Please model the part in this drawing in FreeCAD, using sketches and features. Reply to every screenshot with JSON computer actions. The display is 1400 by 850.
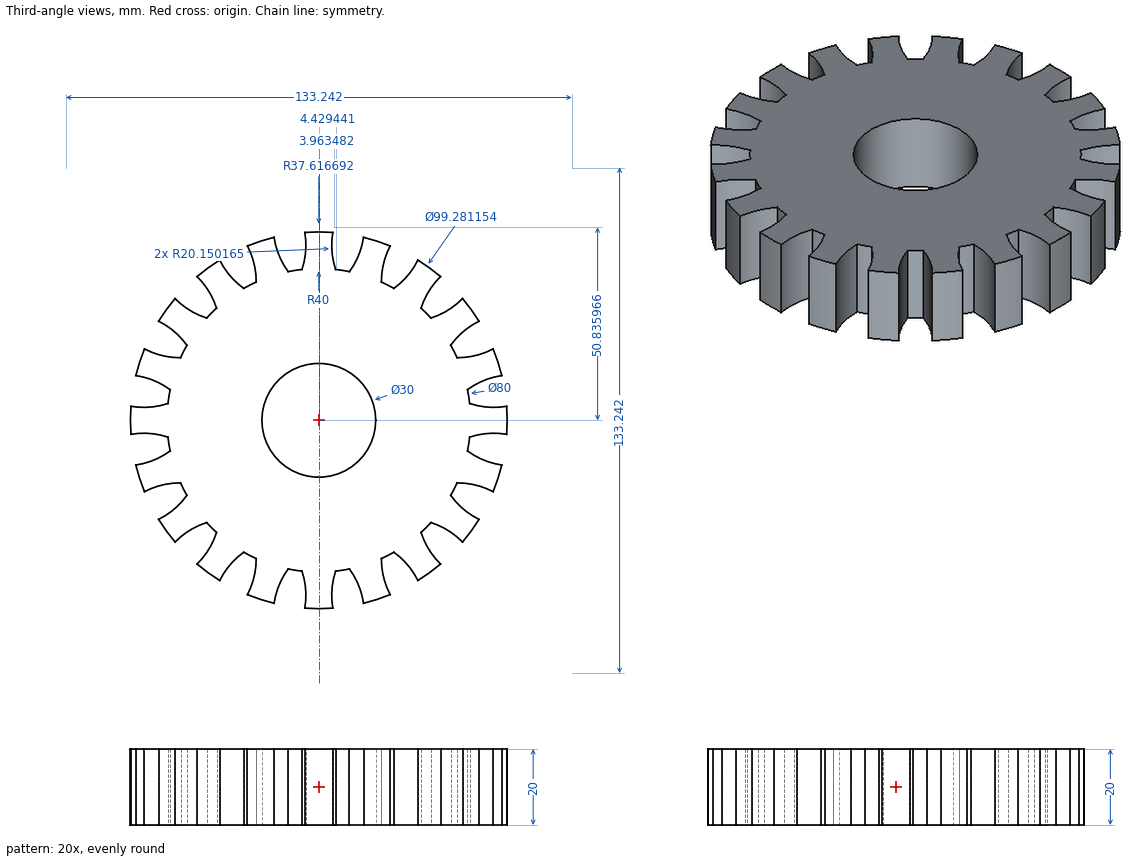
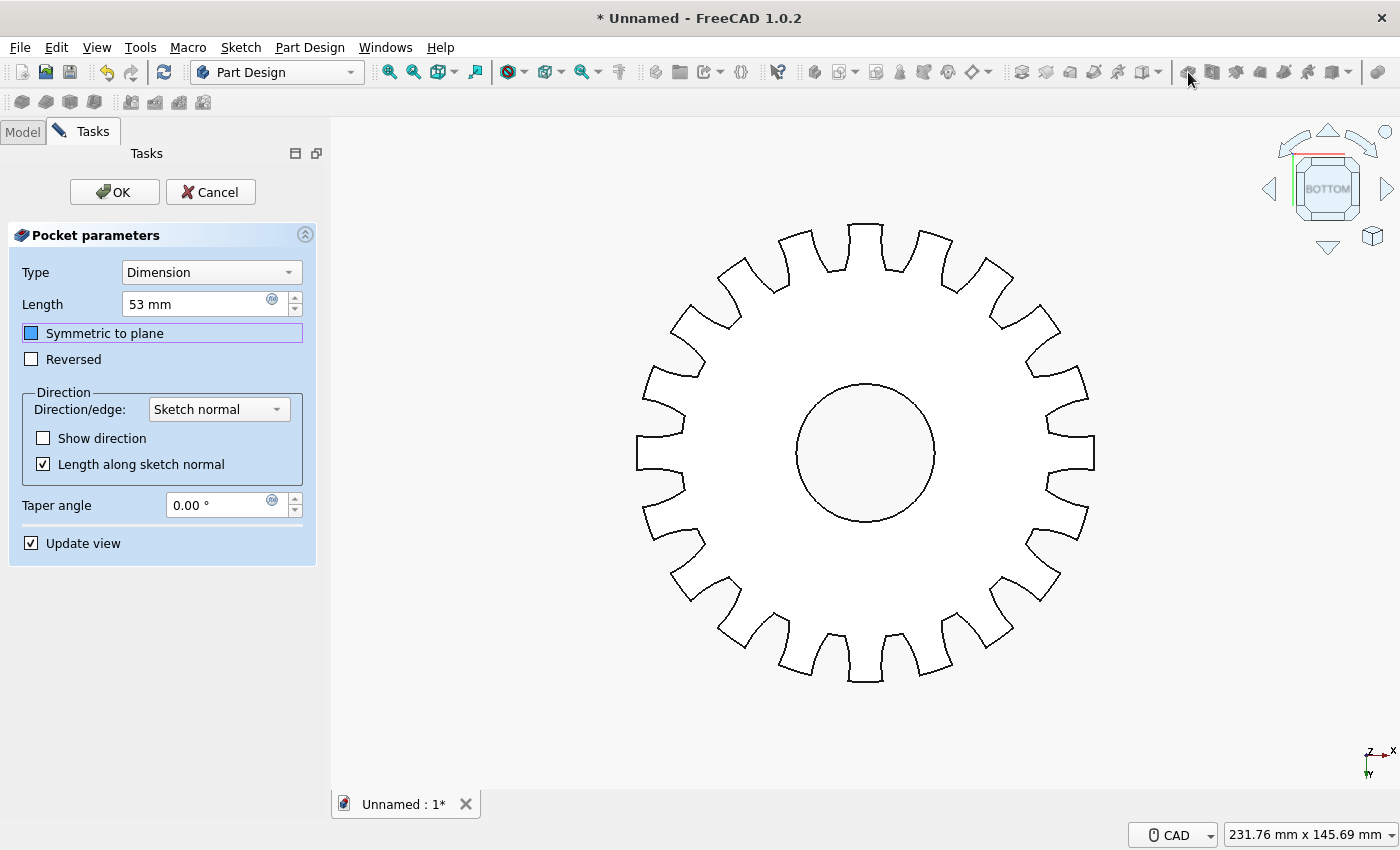
{"action": "left_click", "coordinate": [115, 192]}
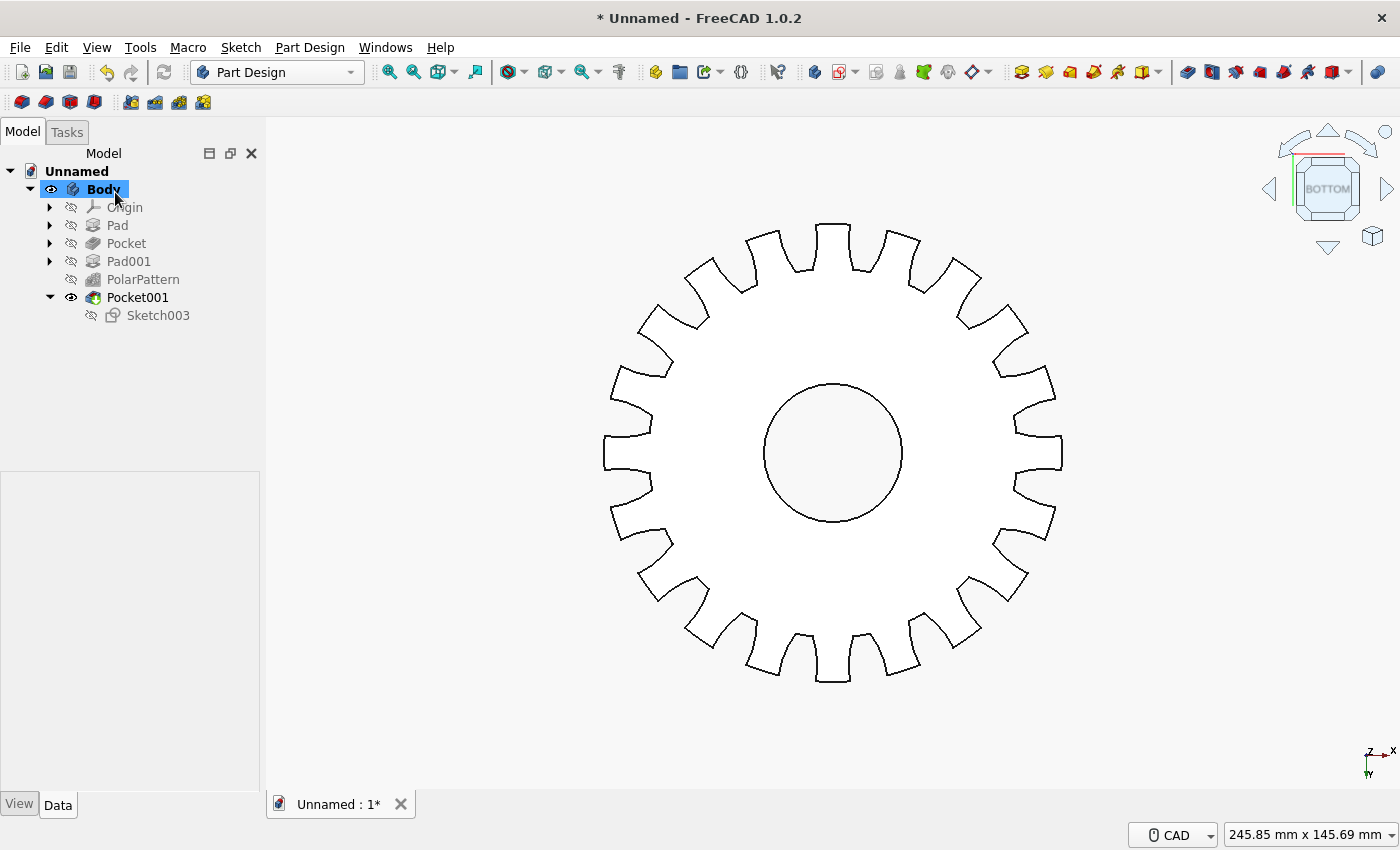
{"action": "key", "text": "0"}